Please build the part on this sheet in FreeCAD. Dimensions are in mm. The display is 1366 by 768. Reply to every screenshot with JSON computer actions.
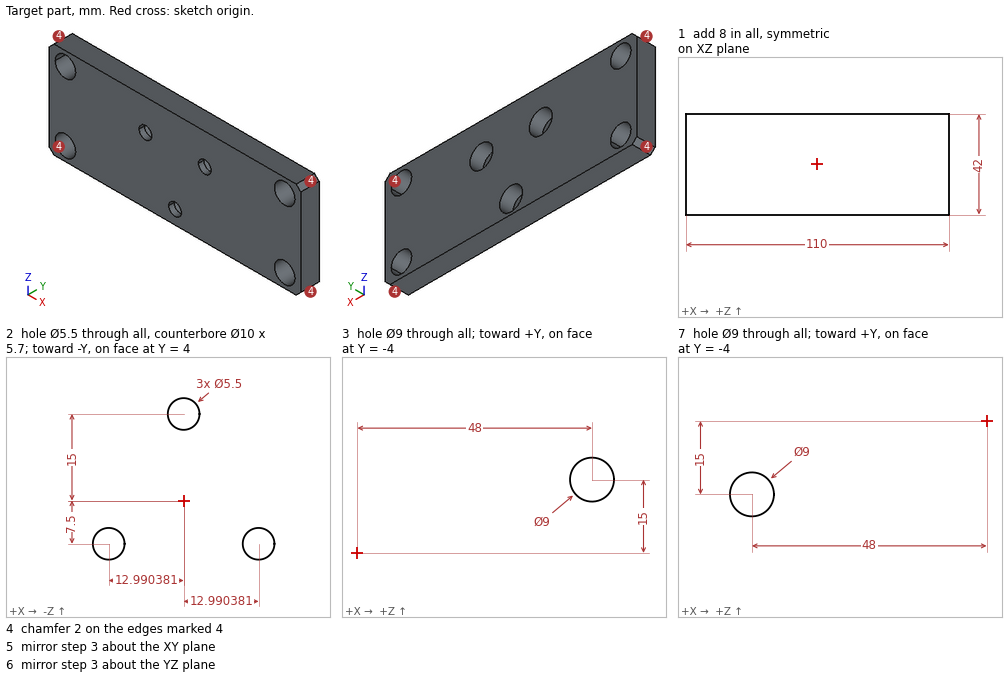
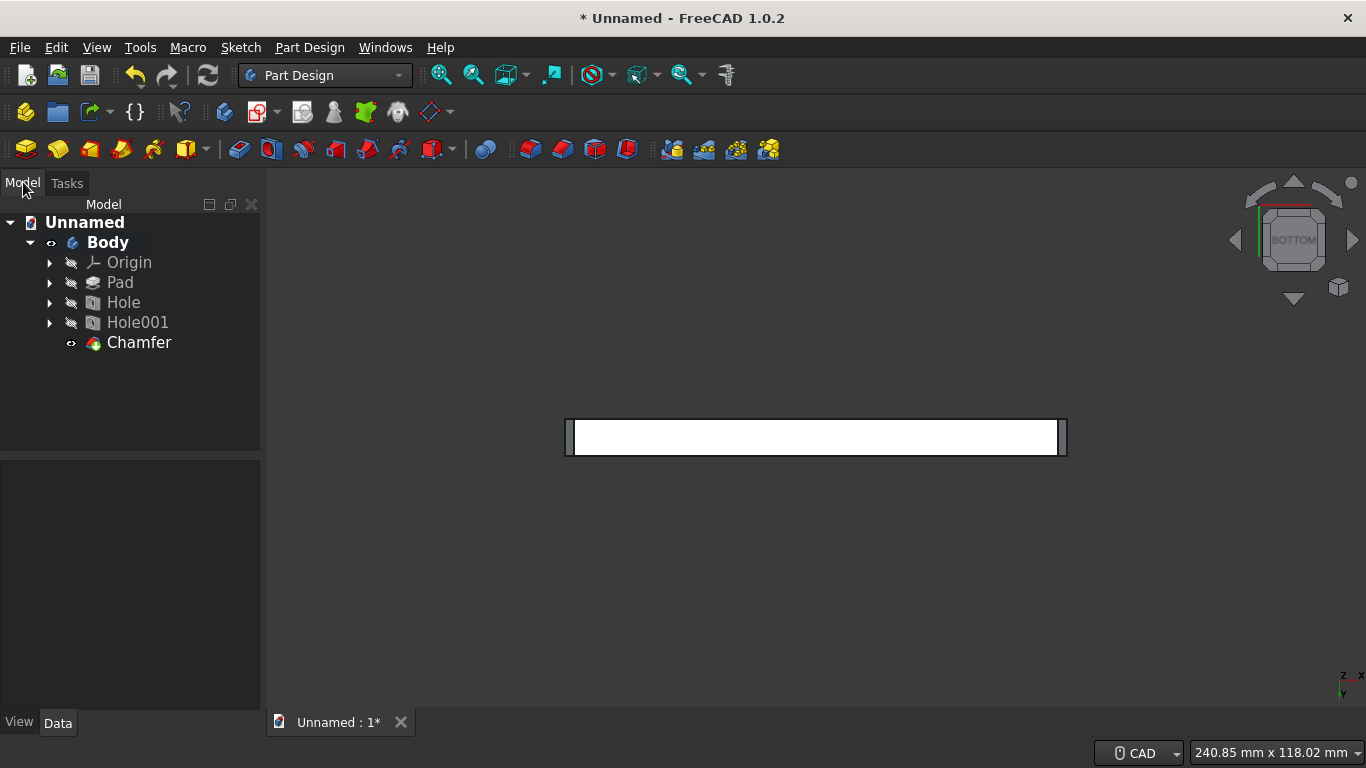
{"action": "left_click", "coordinate": [116, 323]}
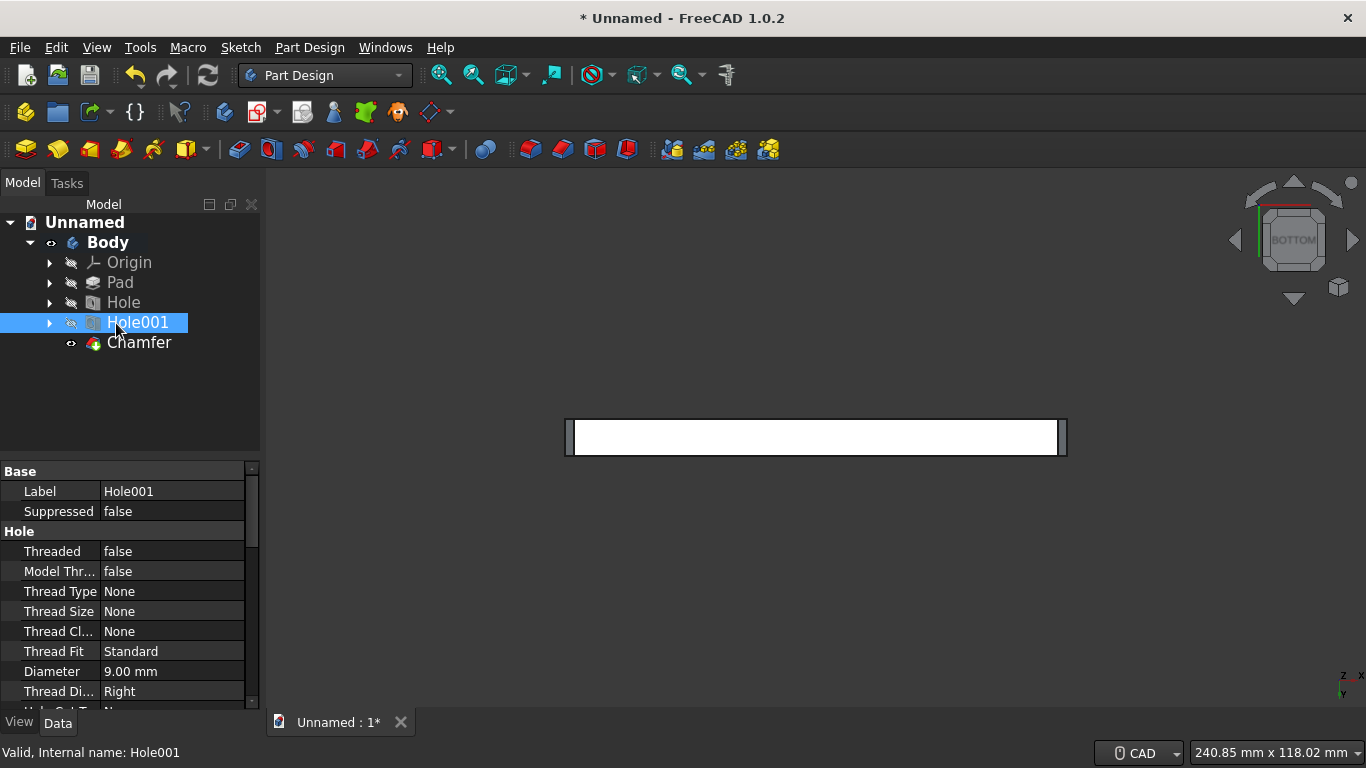
{"action": "left_click", "coordinate": [672, 150]}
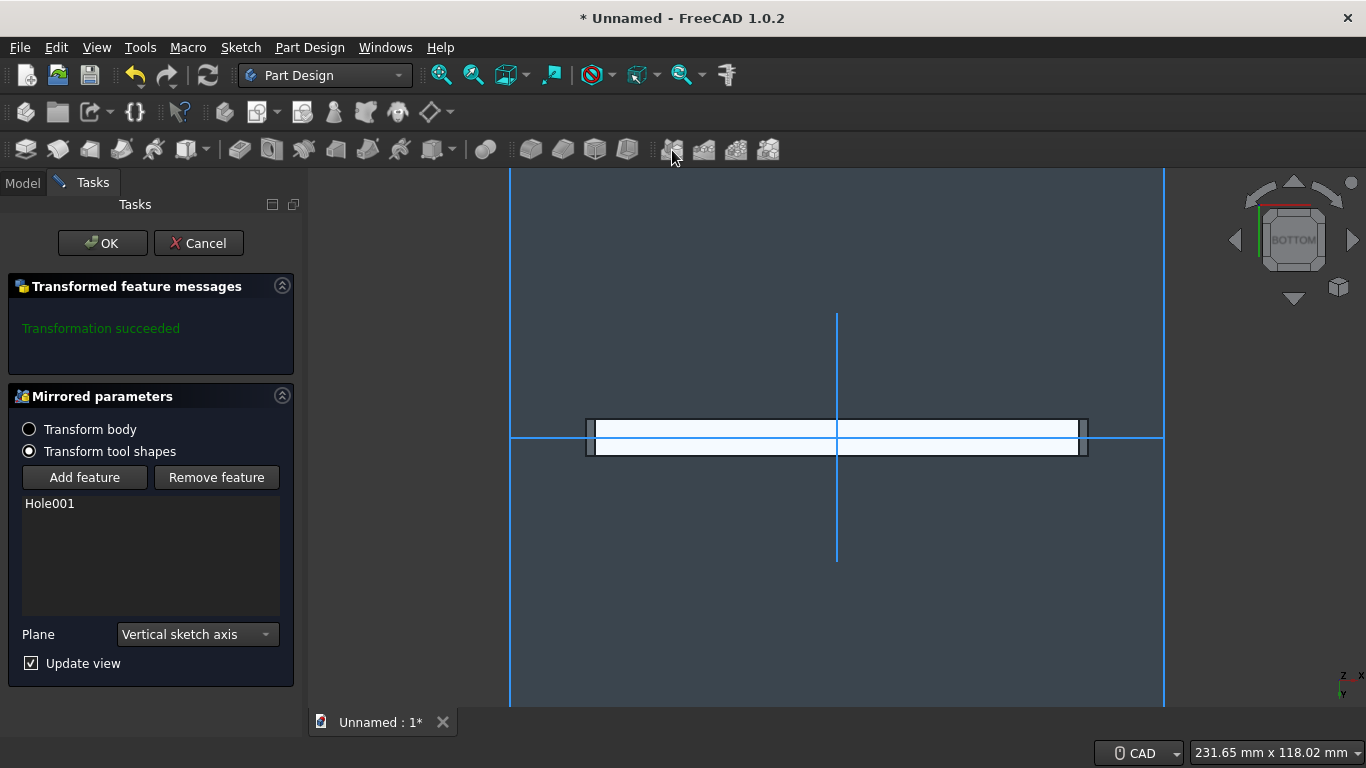
{"action": "left_click", "coordinate": [198, 634]}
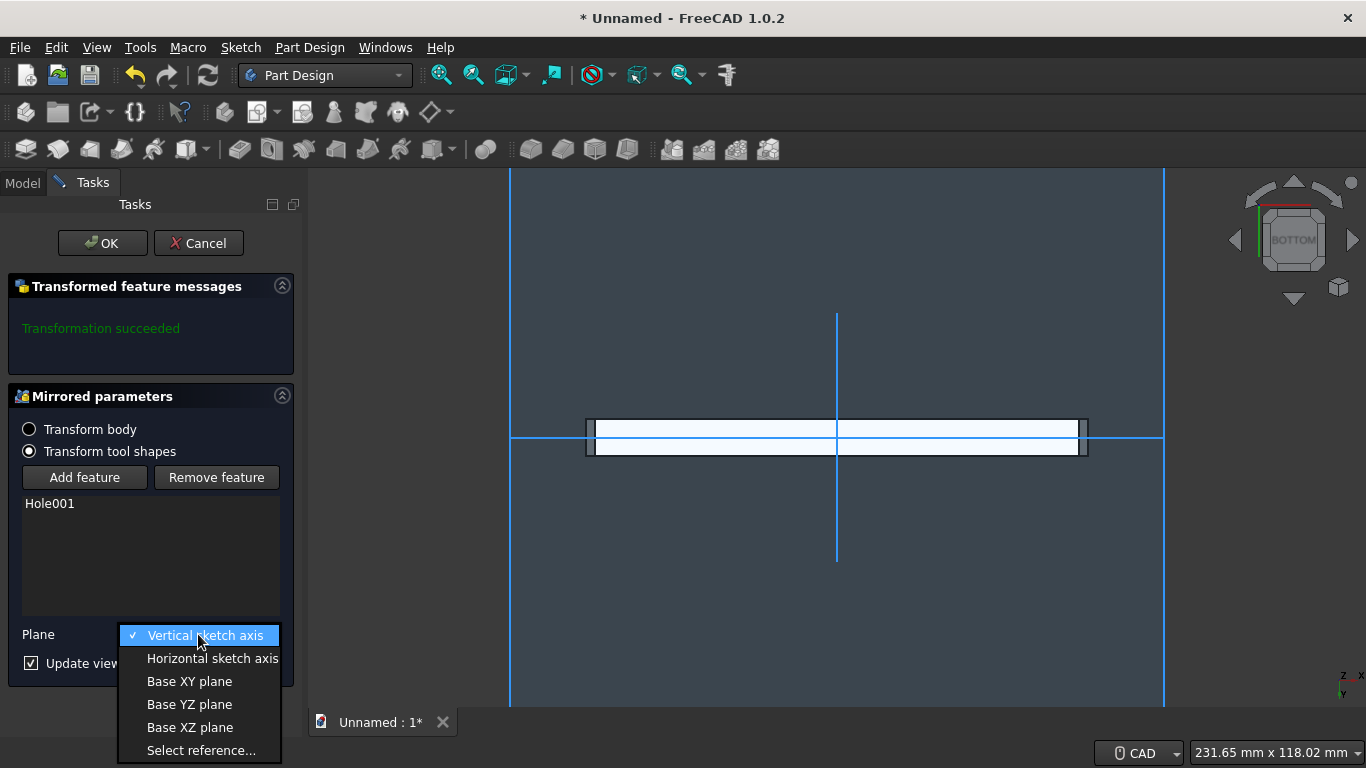
{"action": "left_click", "coordinate": [198, 682]}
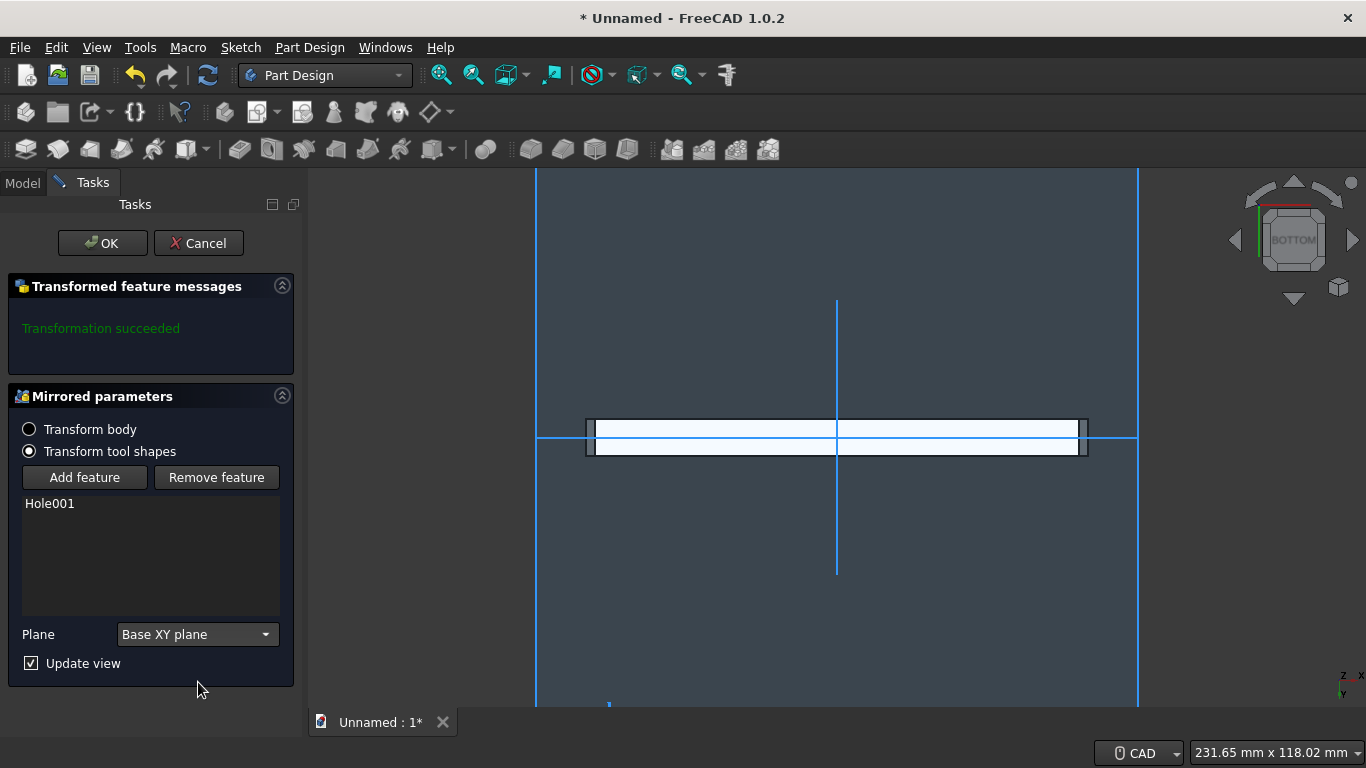
{"action": "left_click", "coordinate": [103, 243]}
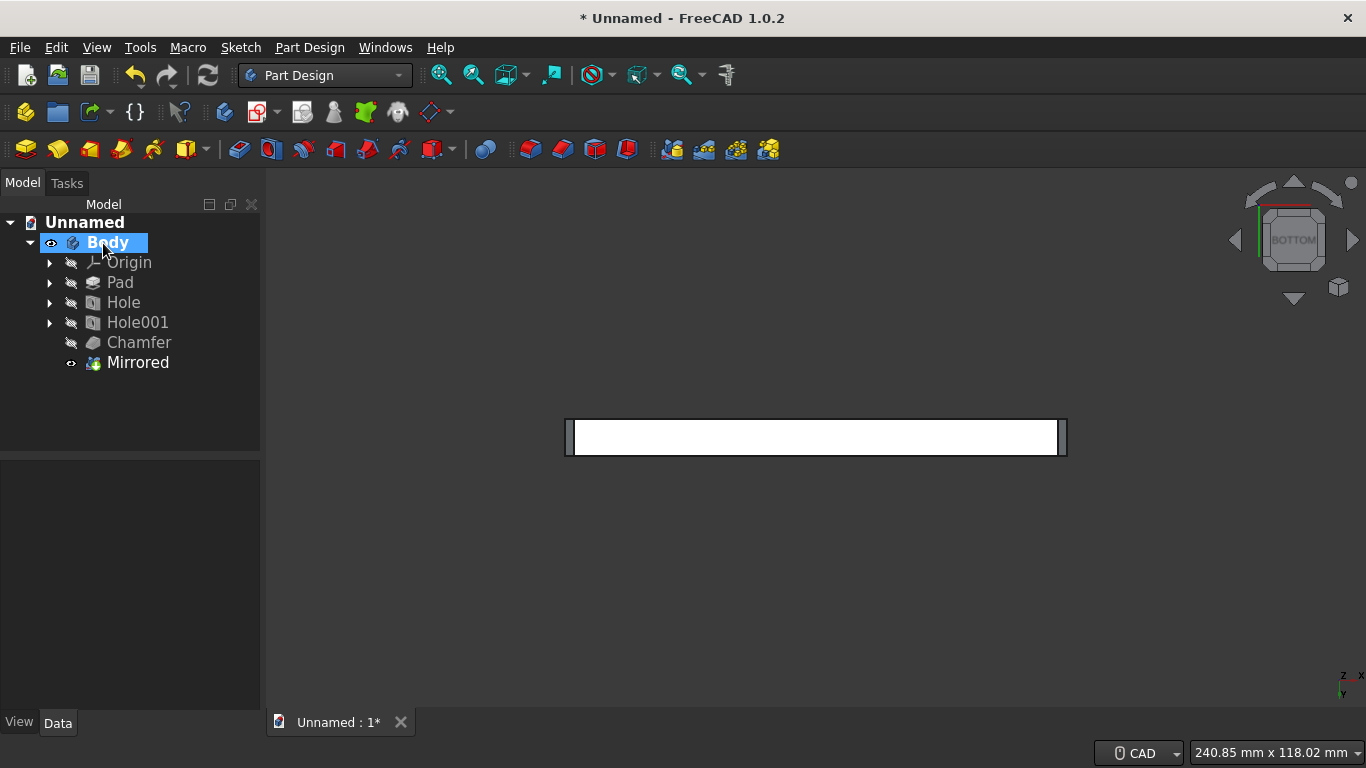
{"action": "left_click", "coordinate": [116, 323]}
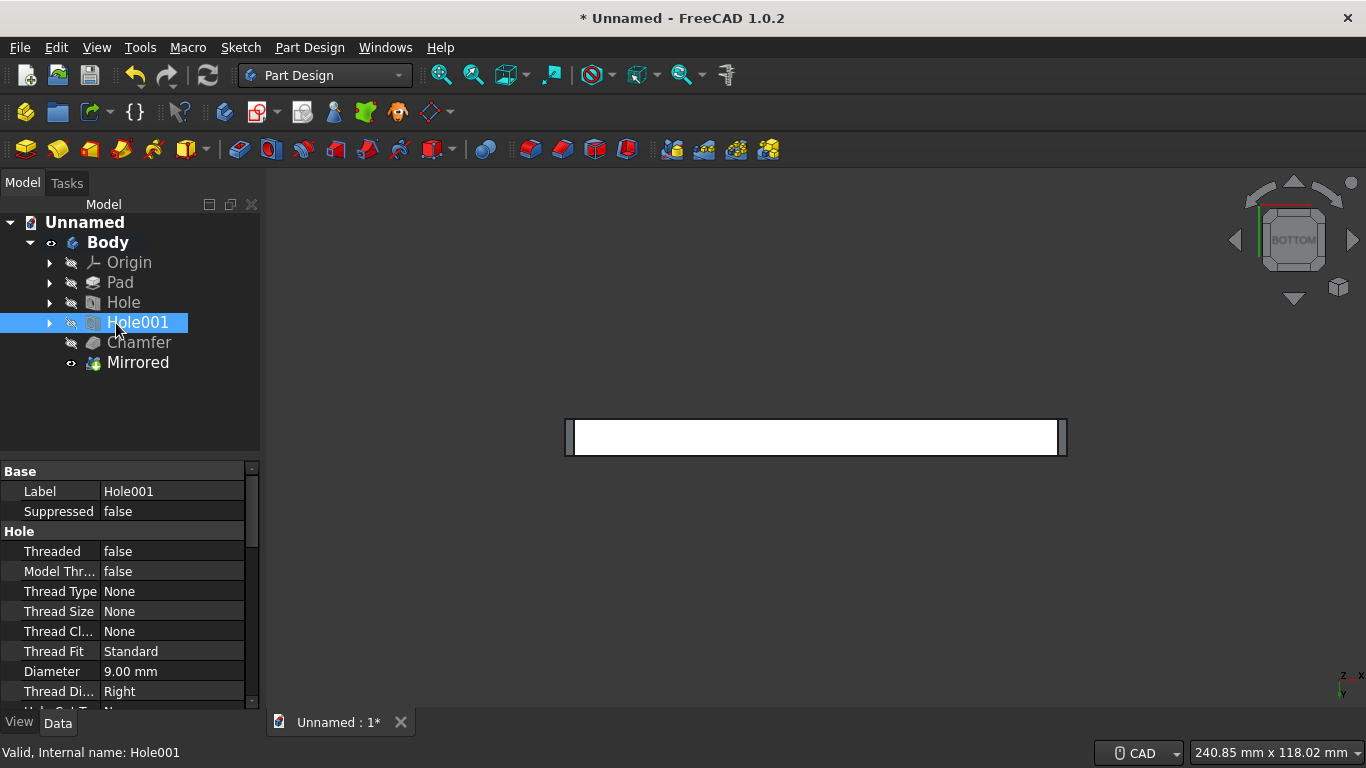
{"action": "left_click", "coordinate": [672, 150]}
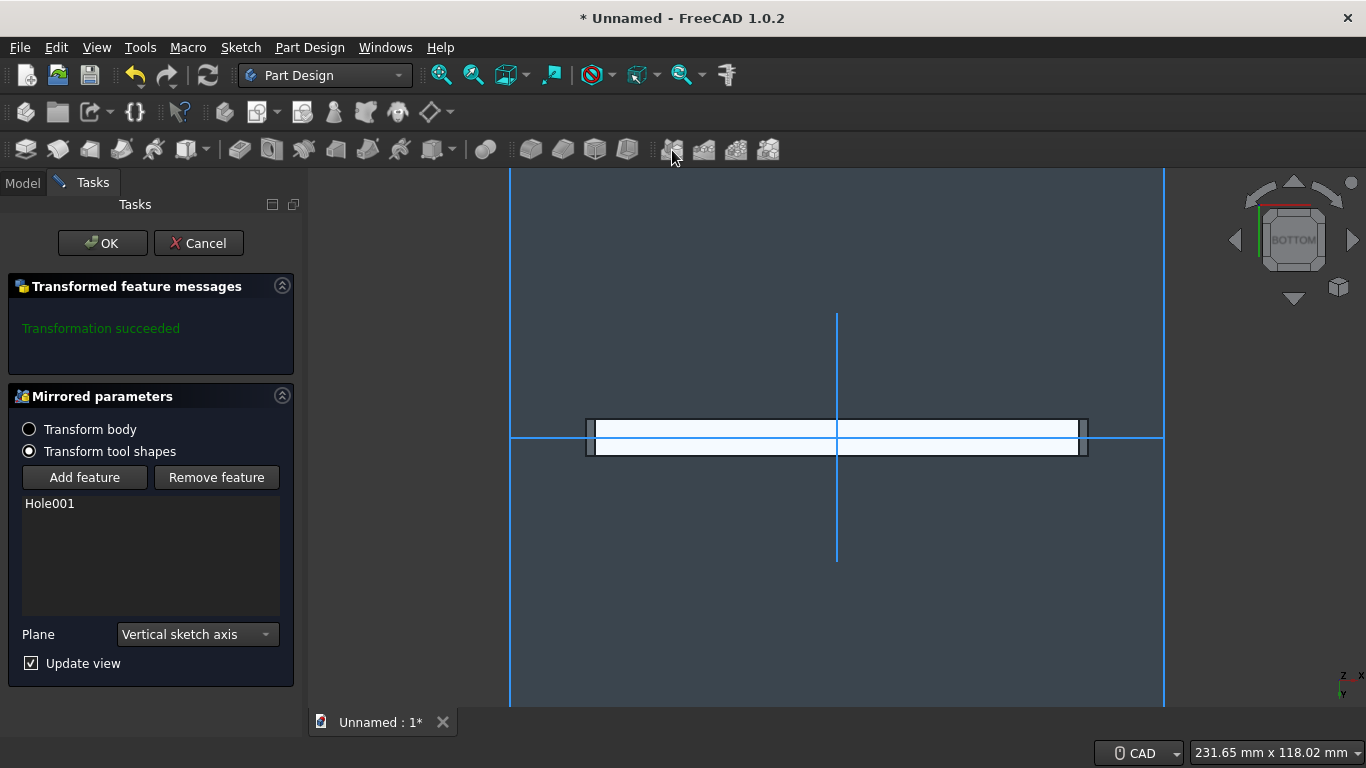
{"action": "left_click", "coordinate": [198, 634]}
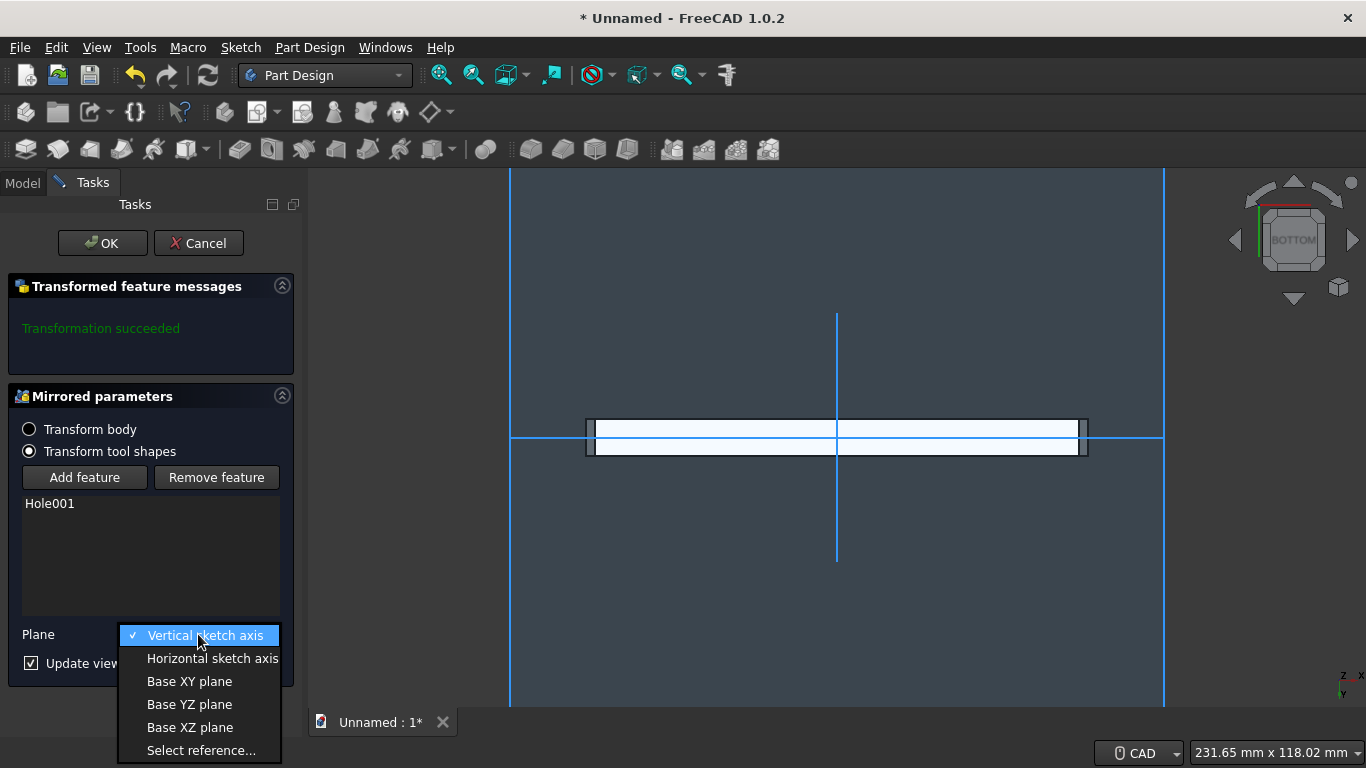
{"action": "left_click", "coordinate": [198, 704]}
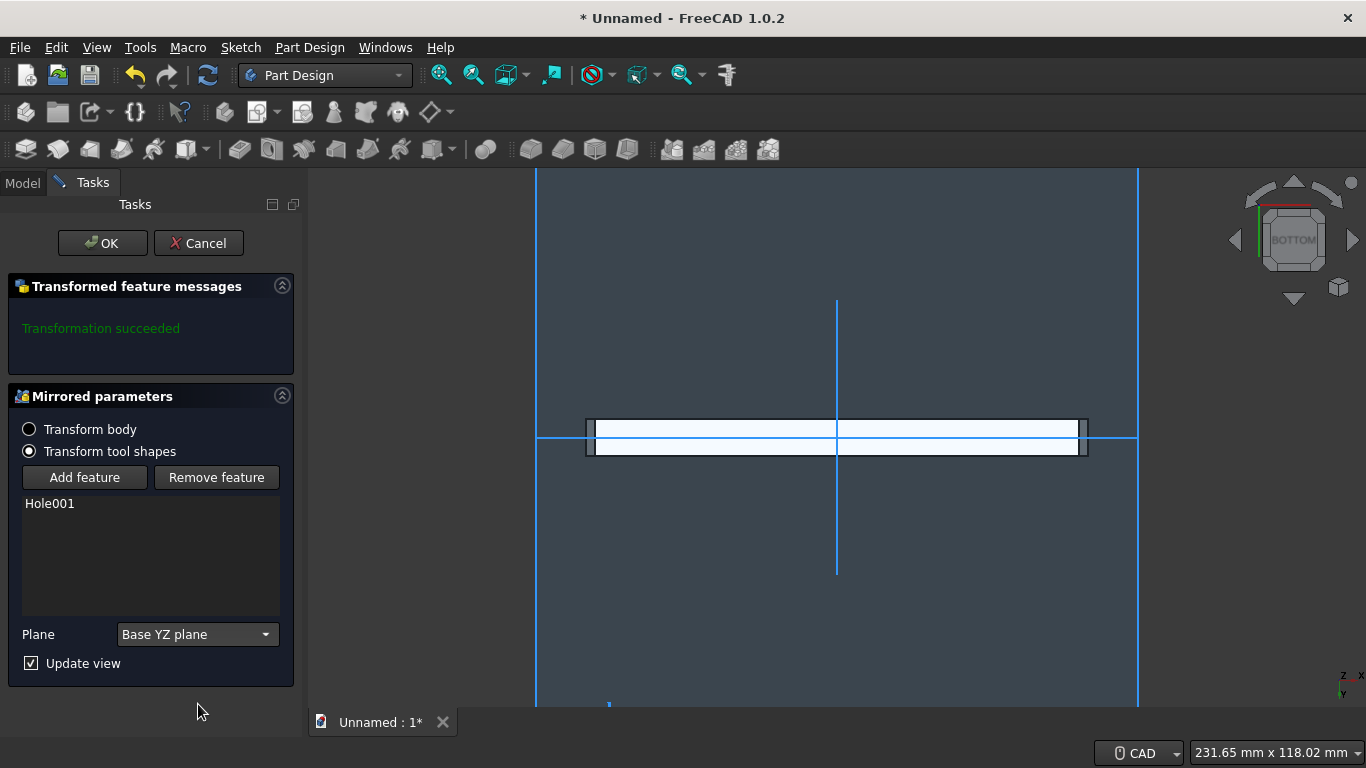
{"action": "left_click", "coordinate": [103, 243]}